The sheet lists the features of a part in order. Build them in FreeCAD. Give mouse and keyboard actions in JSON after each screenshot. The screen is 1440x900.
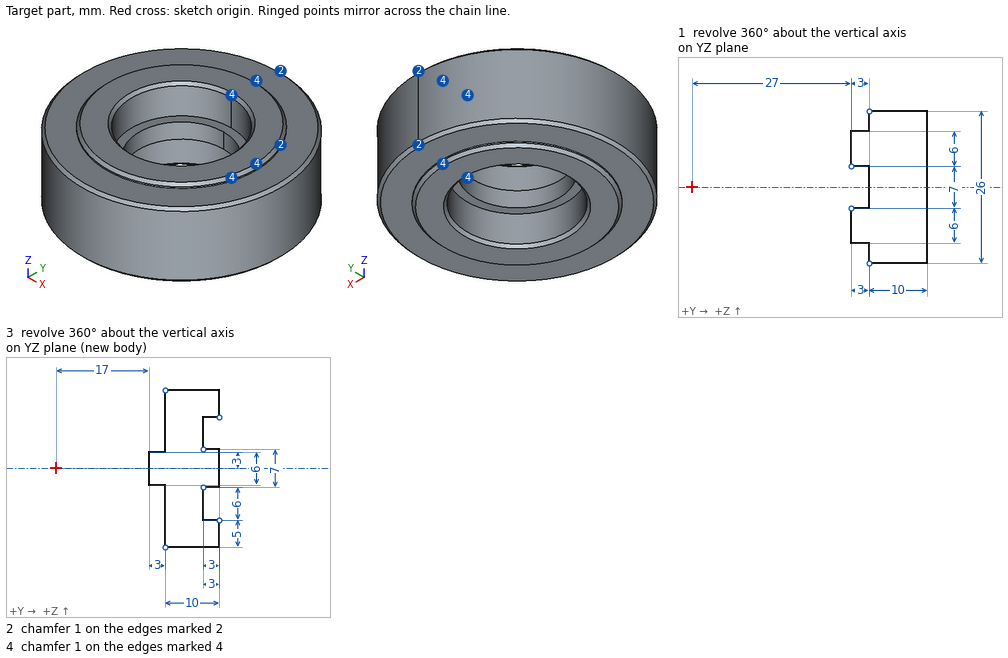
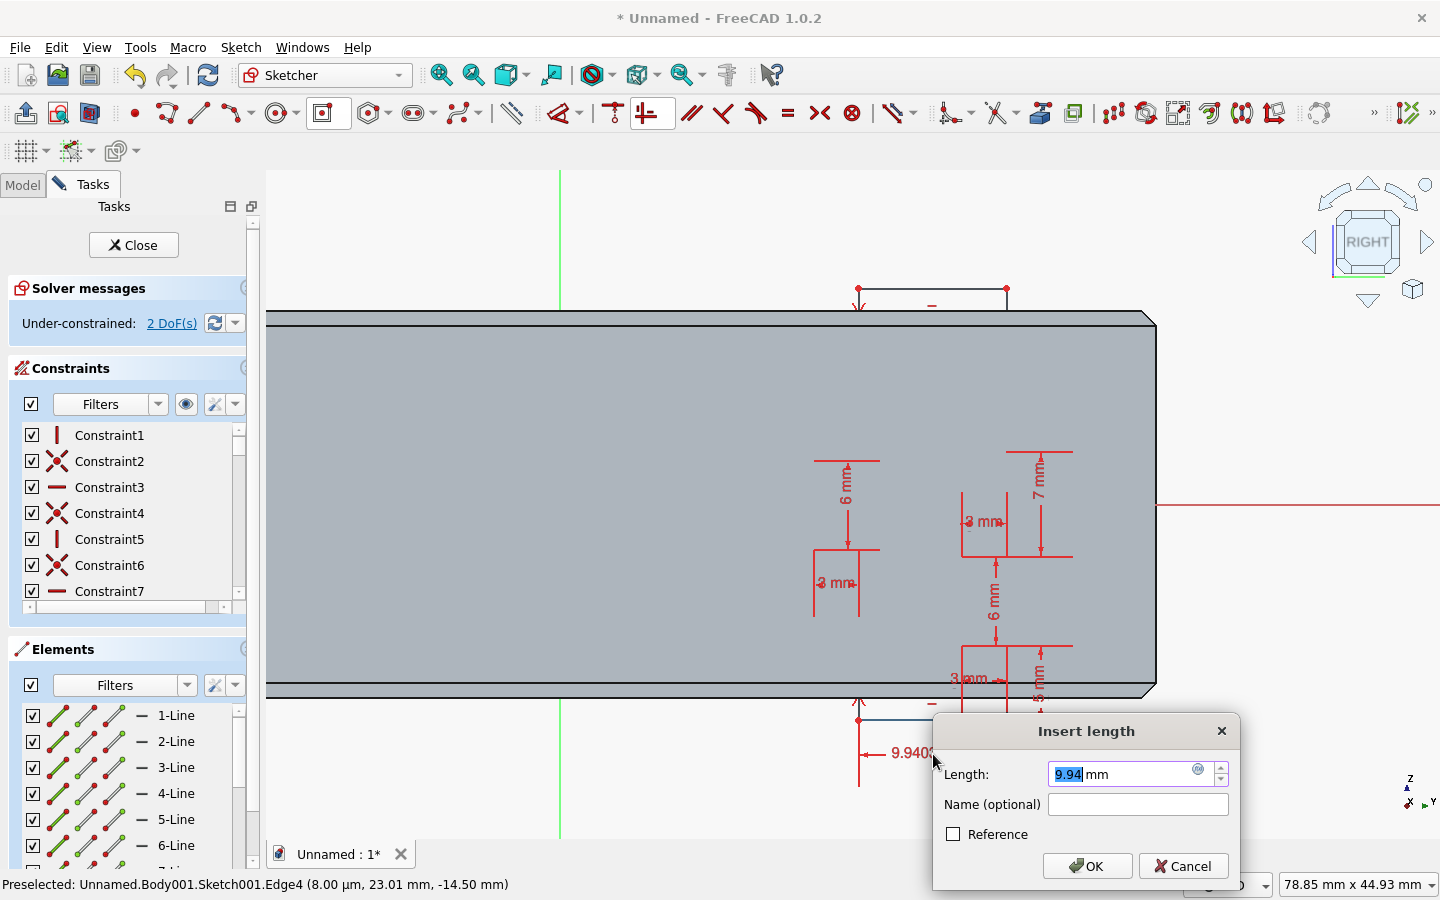
{"action": "type", "text": "10"}
{"action": "key", "text": "Return"}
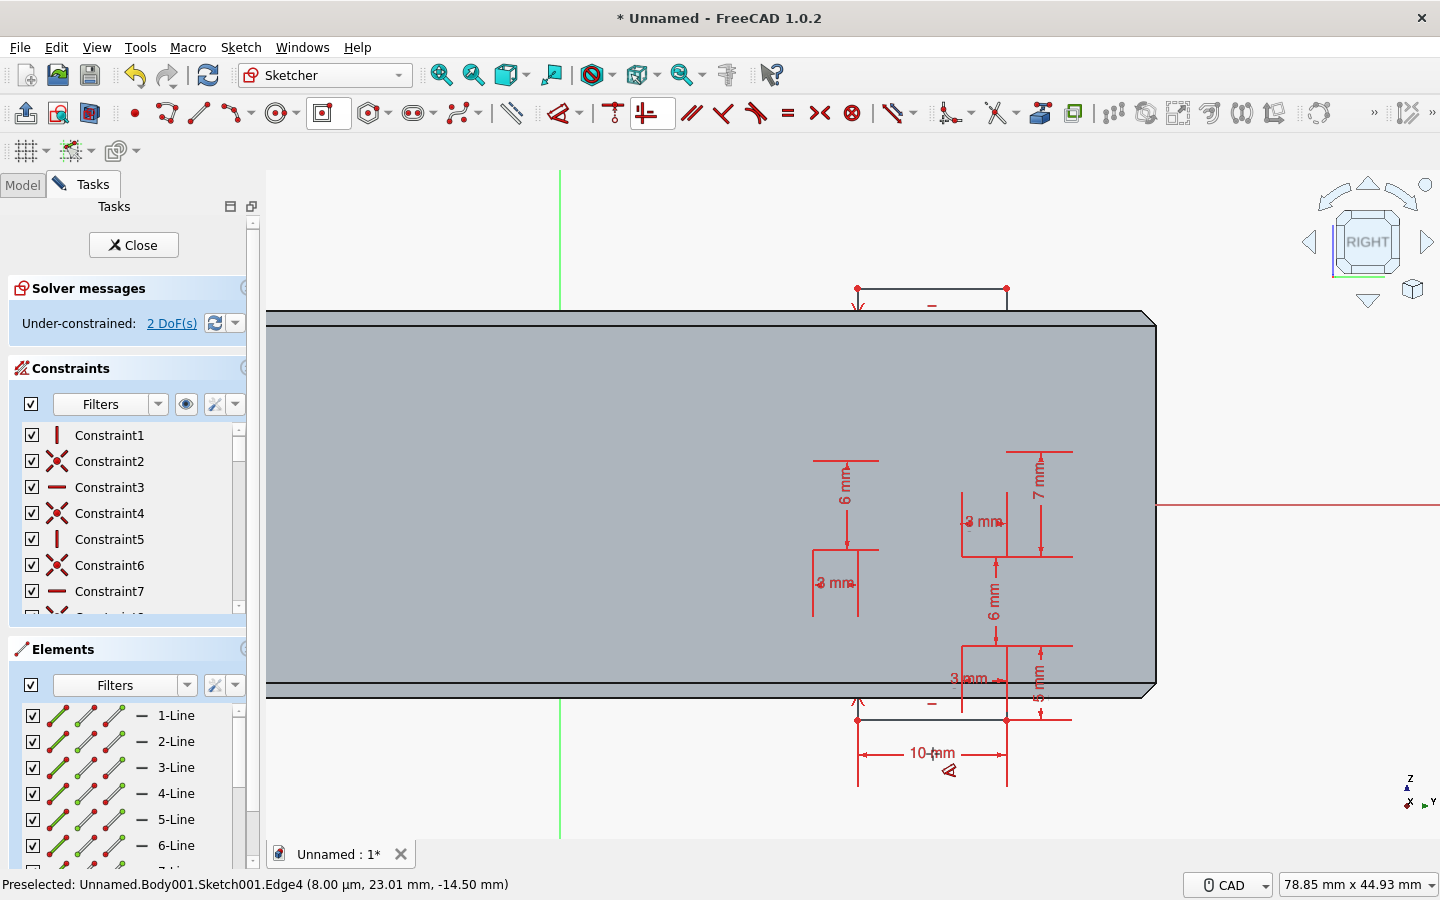
{"action": "left_click", "coordinate": [813, 461]}
{"action": "left_click", "coordinate": [526, 483]}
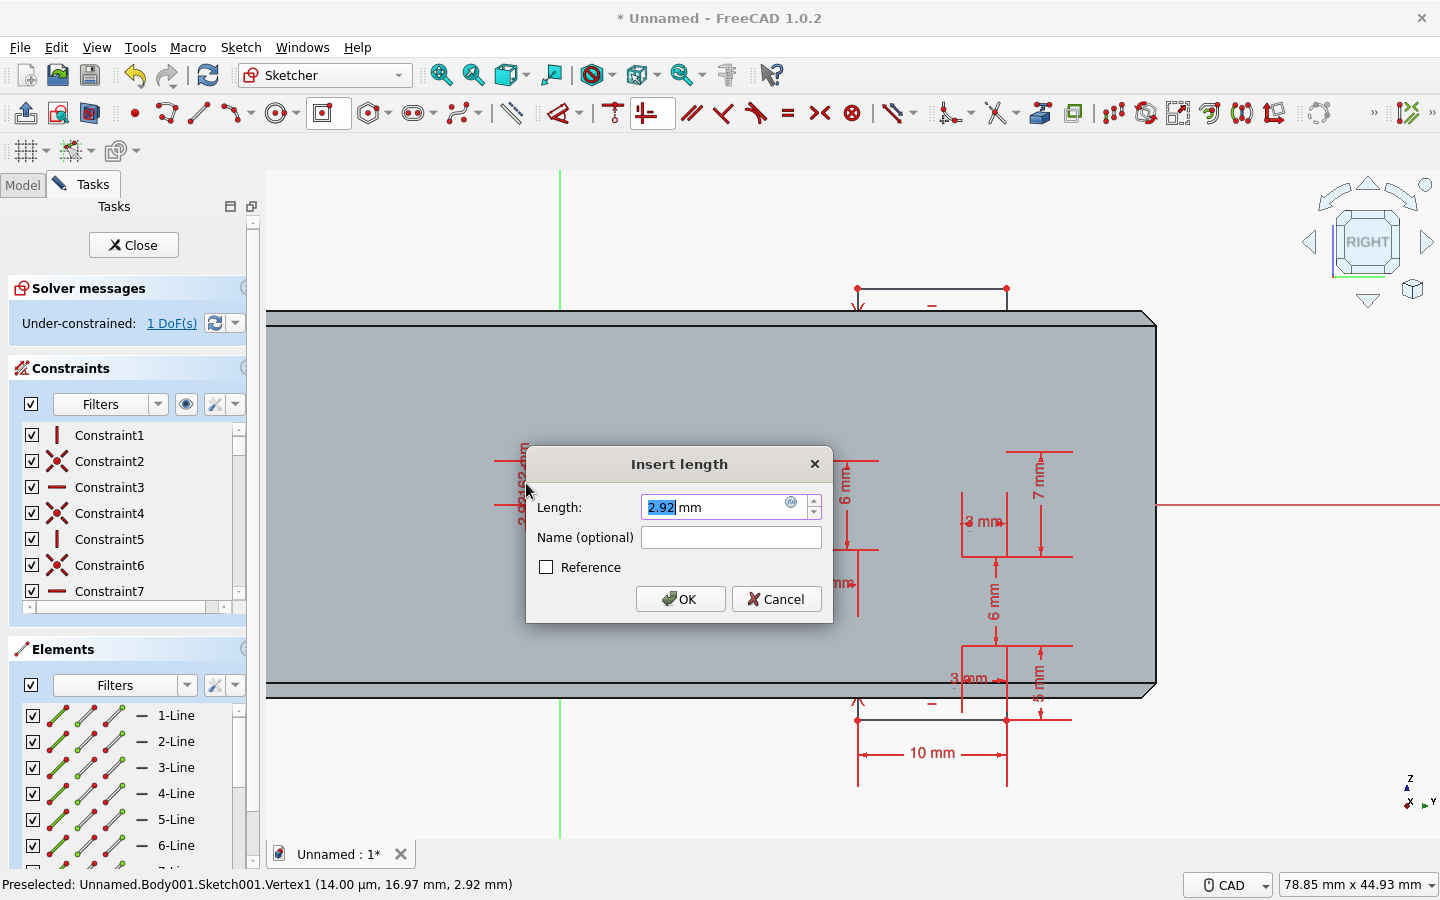
{"action": "type", "text": "3"}
{"action": "key", "text": "Return"}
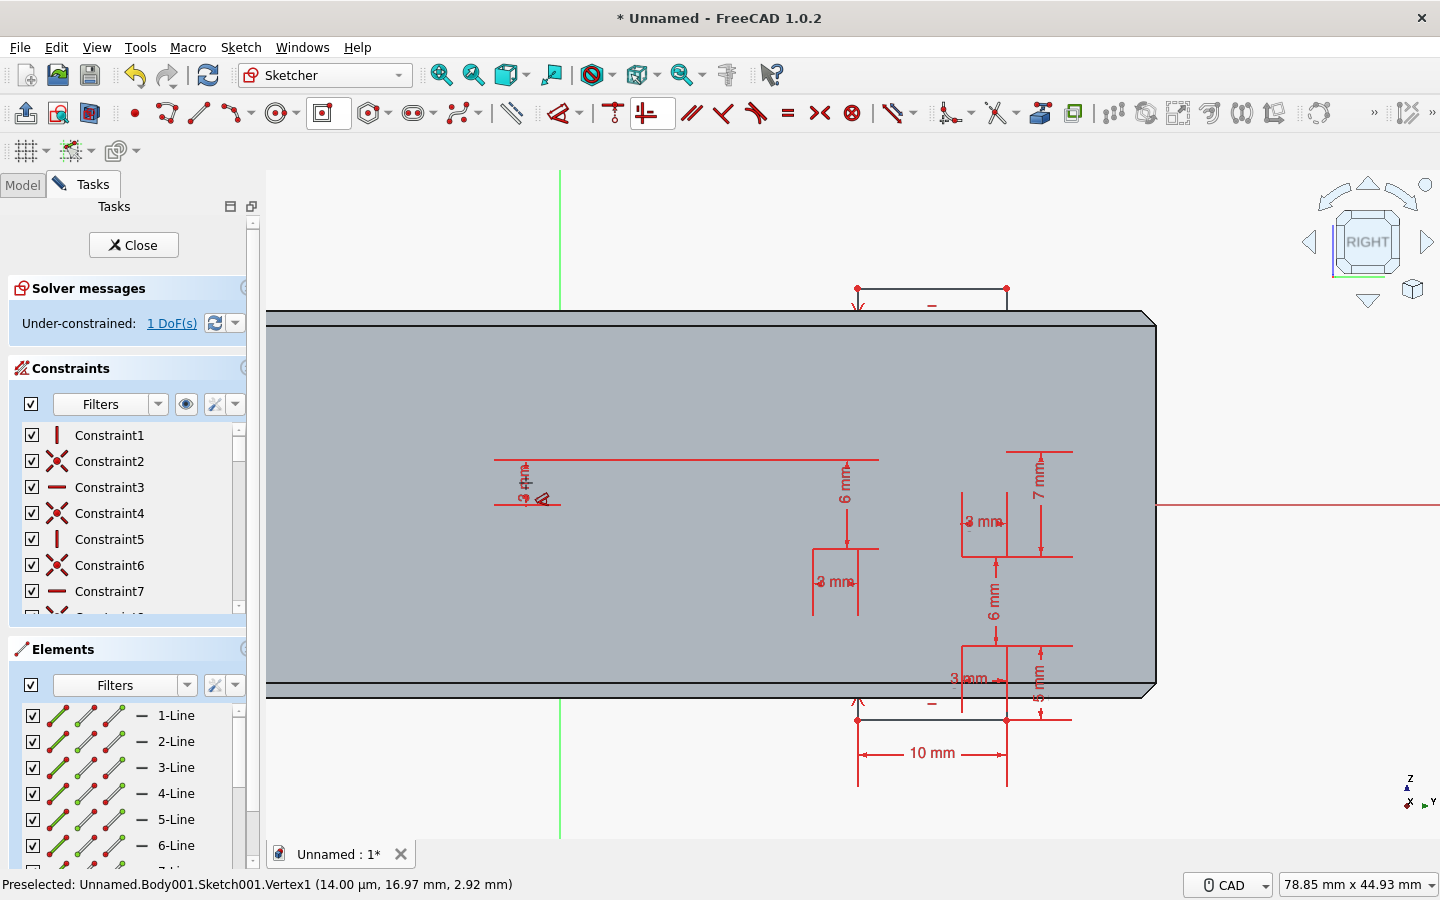
{"action": "left_click", "coordinate": [813, 460]}
{"action": "left_click", "coordinate": [687, 426]}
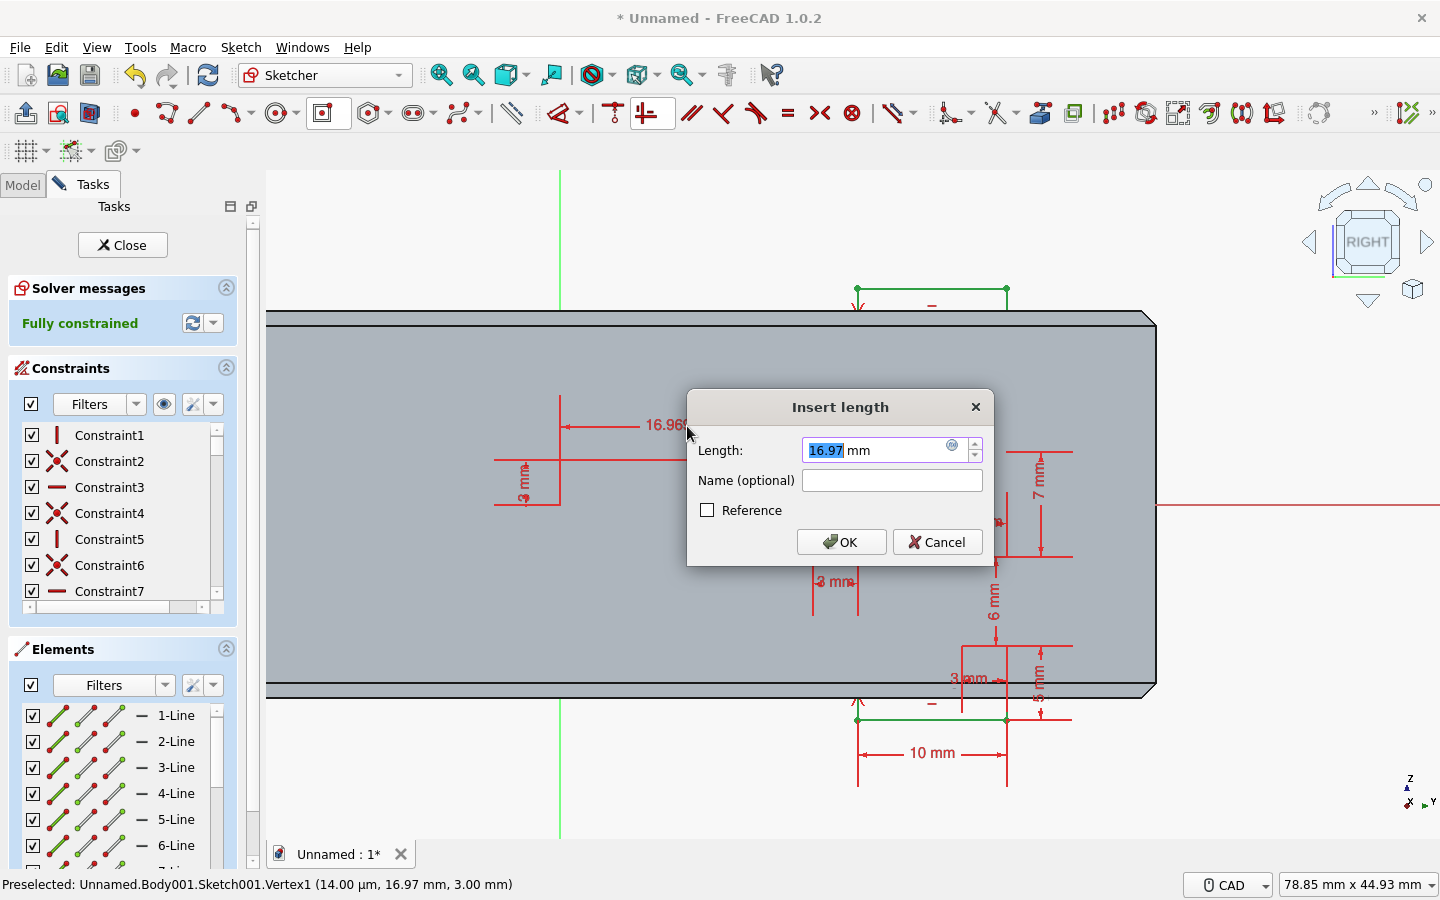
{"action": "type", "text": "17"}
{"action": "key", "text": "Return"}
{"action": "key", "text": "Escape"}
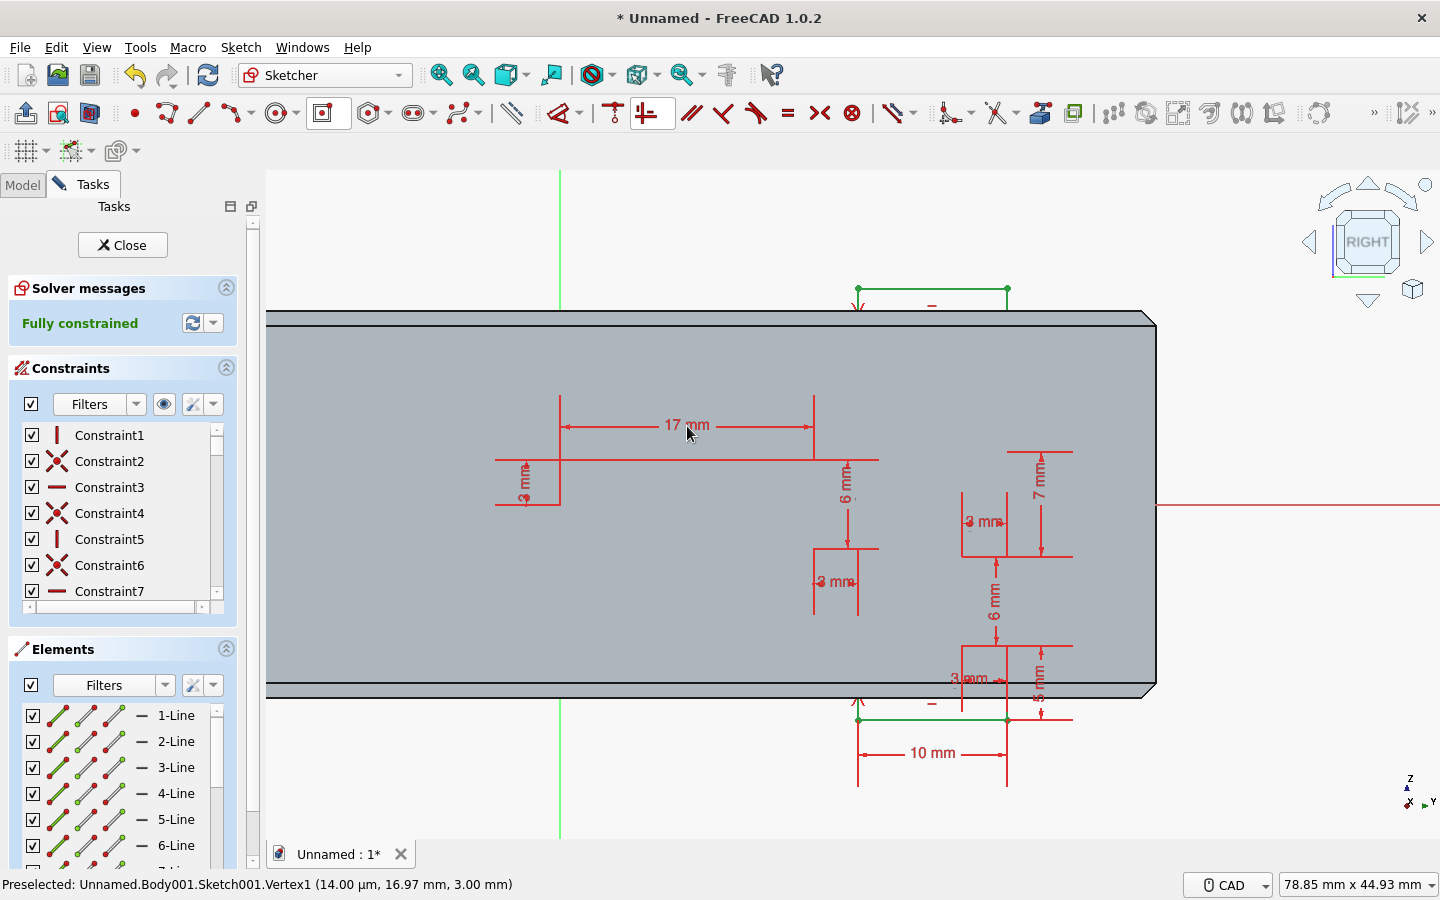
{"action": "left_click", "coordinate": [123, 245]}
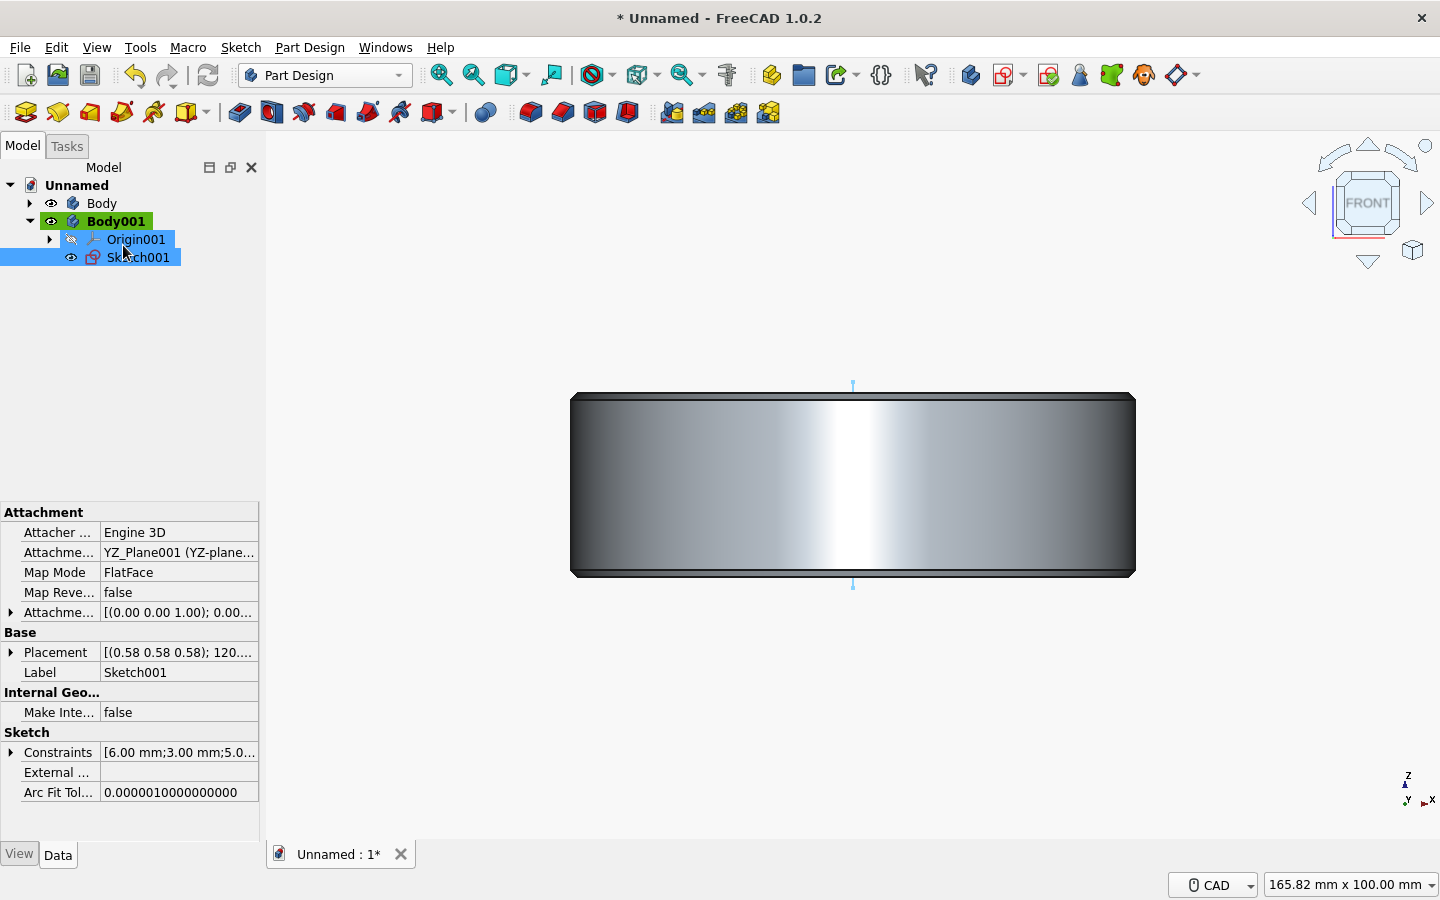
{"action": "left_click", "coordinate": [58, 112]}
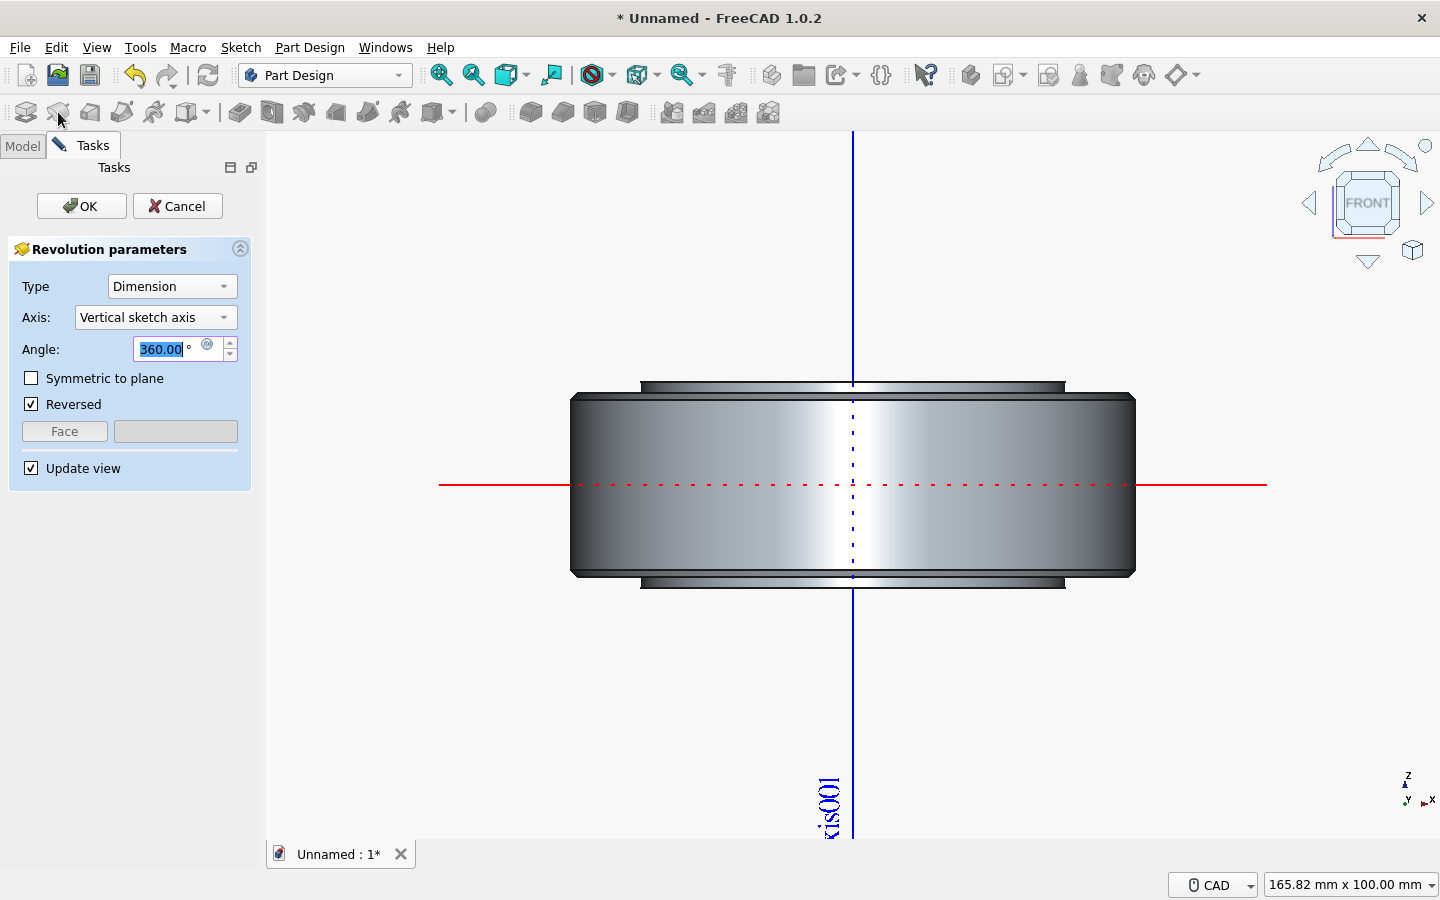
{"action": "left_click", "coordinate": [82, 206]}